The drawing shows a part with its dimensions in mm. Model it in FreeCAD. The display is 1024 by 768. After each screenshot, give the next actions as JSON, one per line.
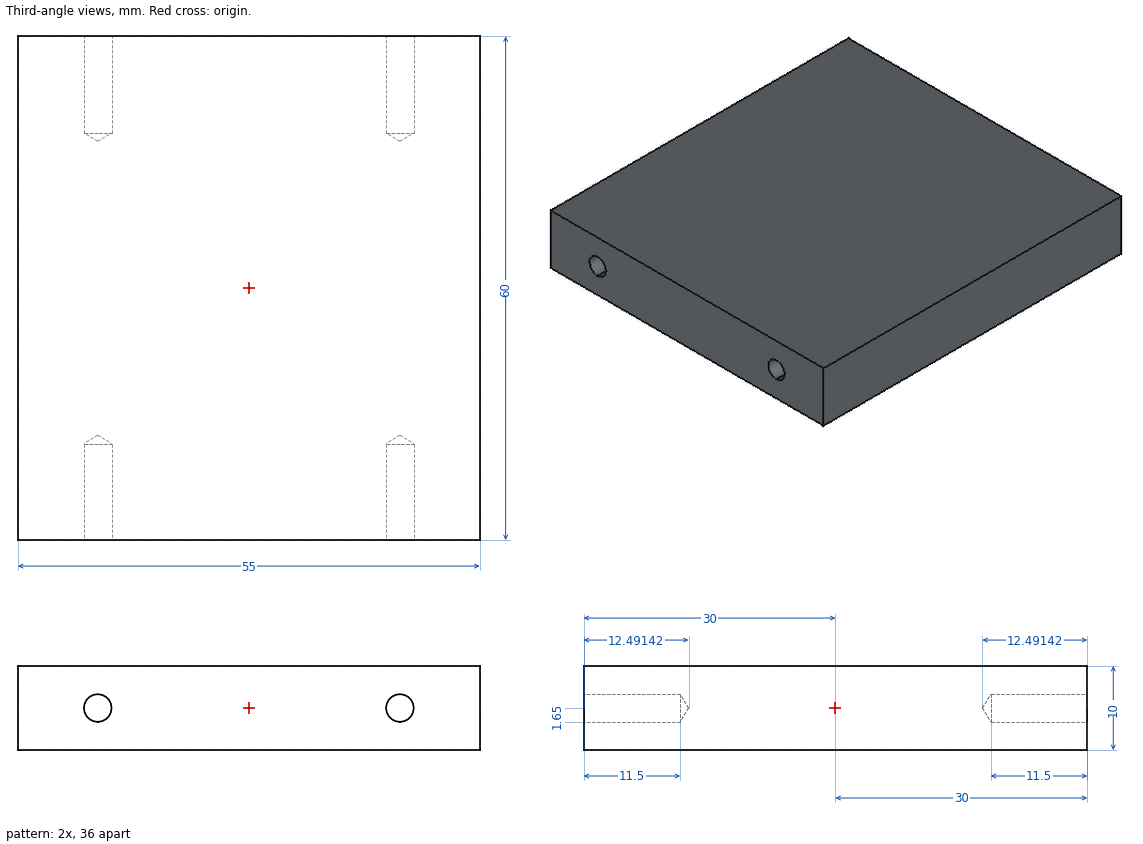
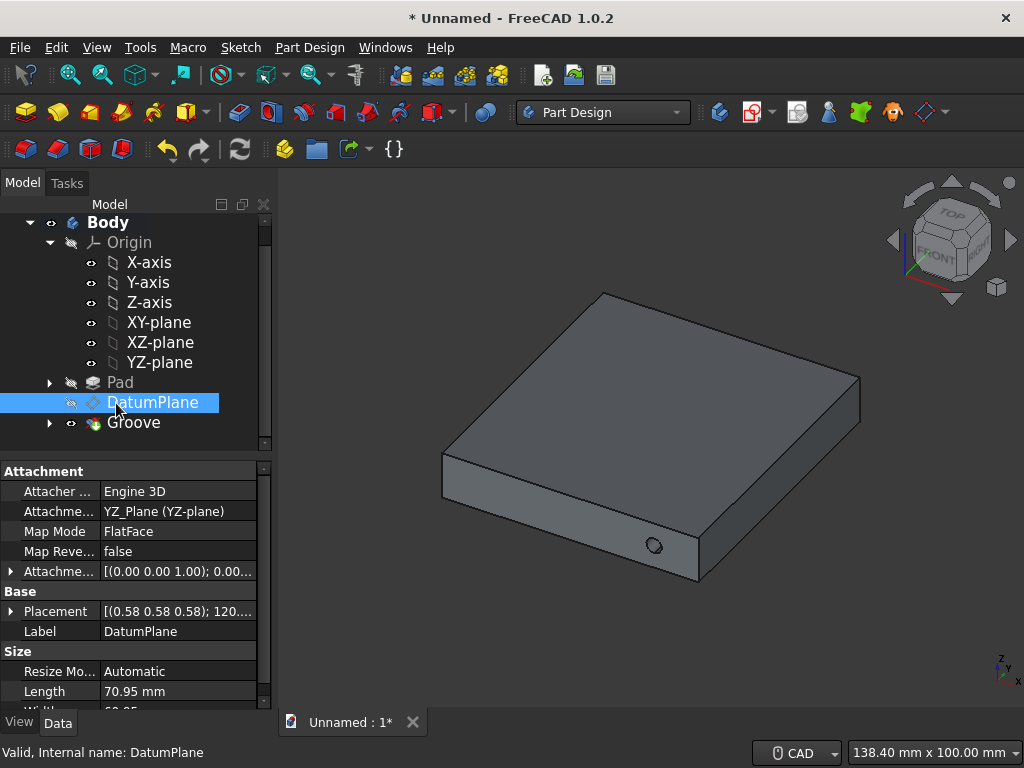
{"action": "left_click", "coordinate": [116, 423]}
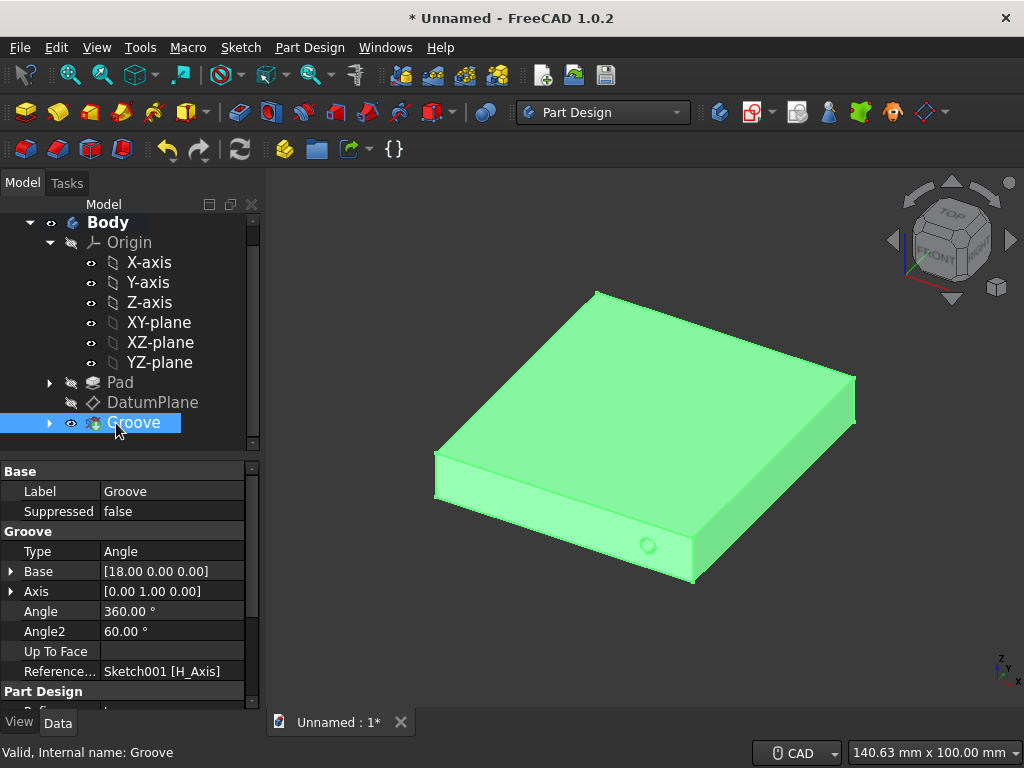
{"action": "left_click", "coordinate": [434, 76]}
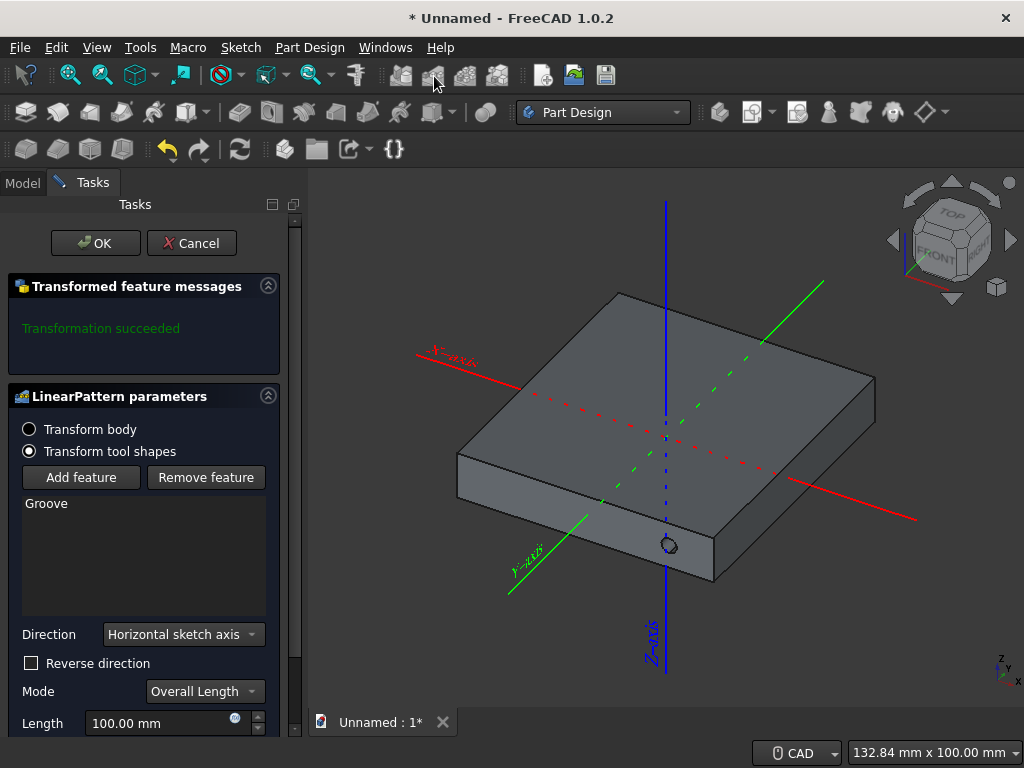
{"action": "left_click", "coordinate": [184, 634]}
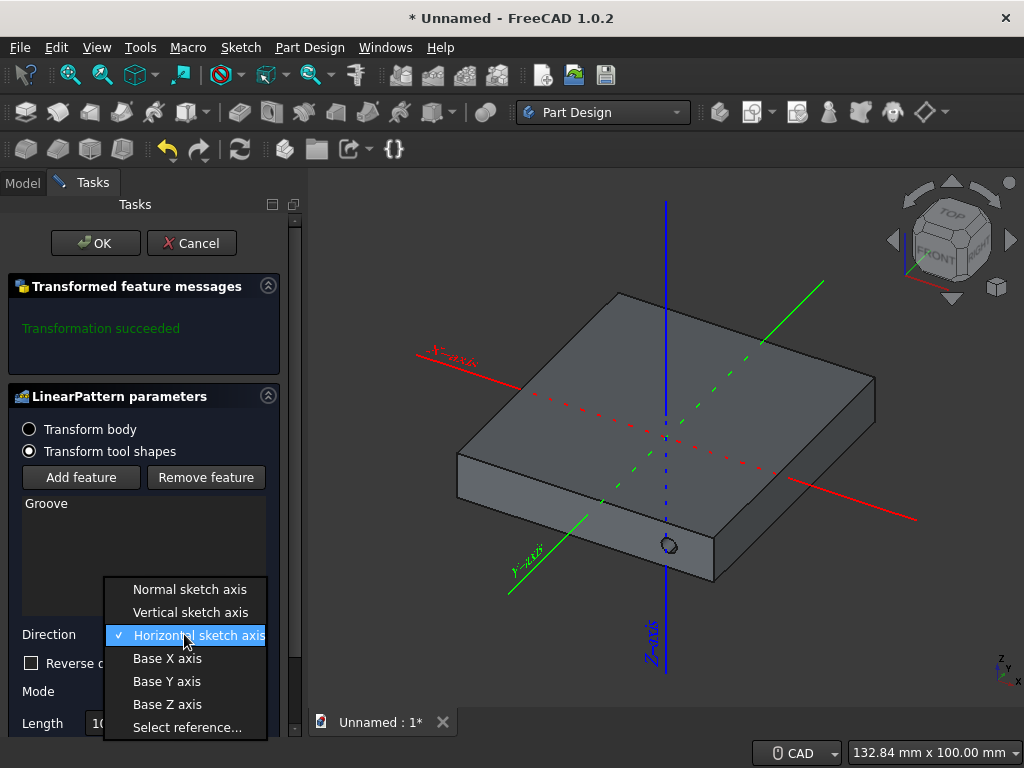
{"action": "left_click", "coordinate": [184, 658]}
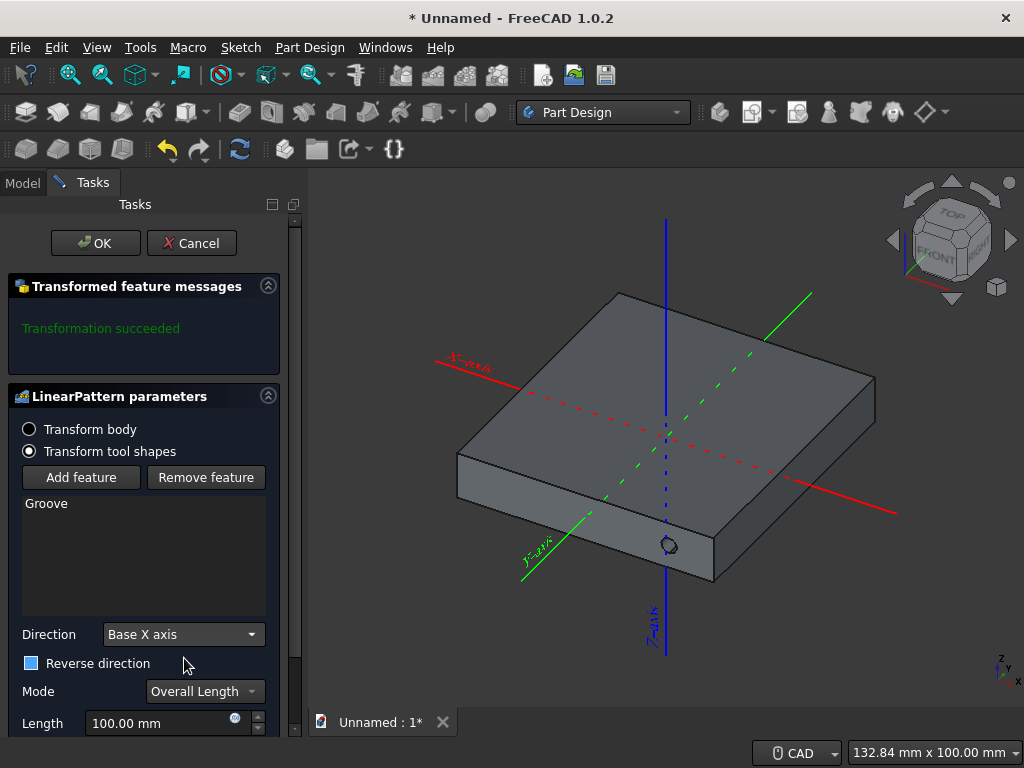
{"action": "left_click", "coordinate": [206, 692]}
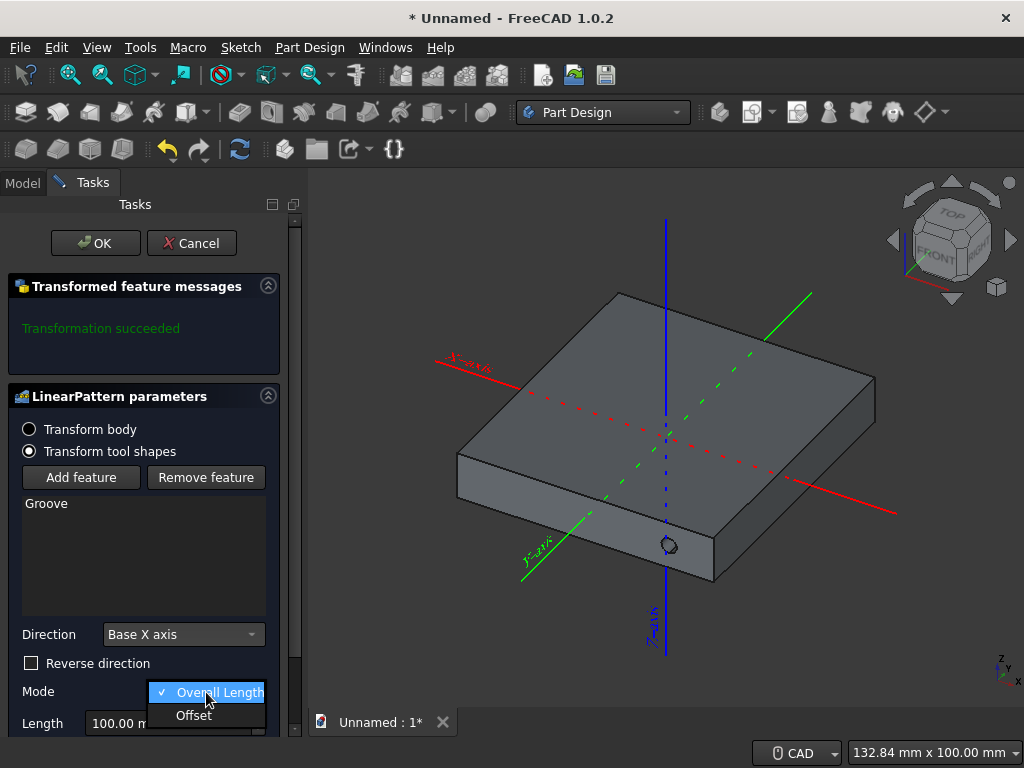
{"action": "left_click", "coordinate": [206, 716]}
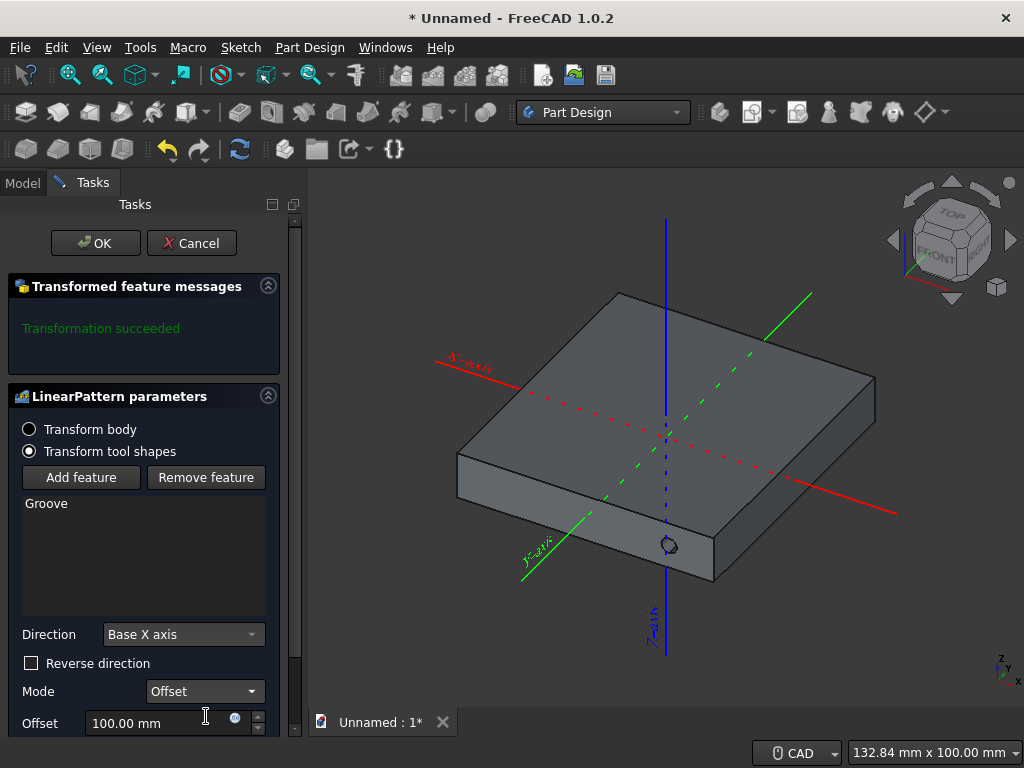
{"action": "triple_click", "coordinate": [168, 723]}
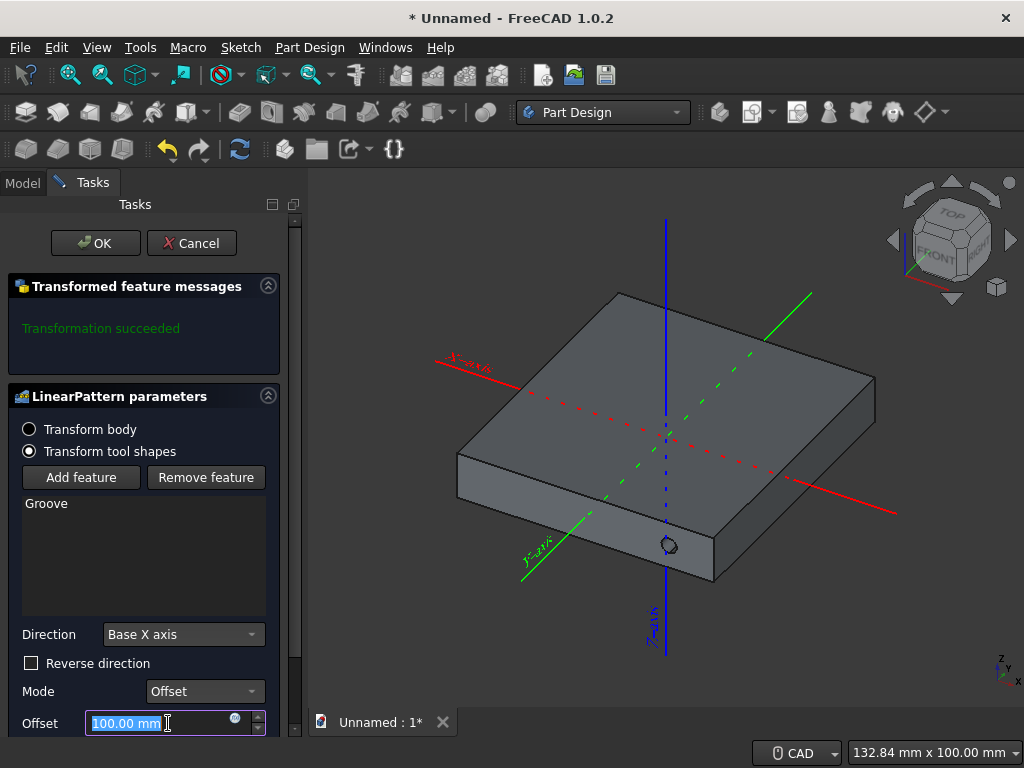
{"action": "type", "text": "36"}
{"action": "key", "text": "Tab"}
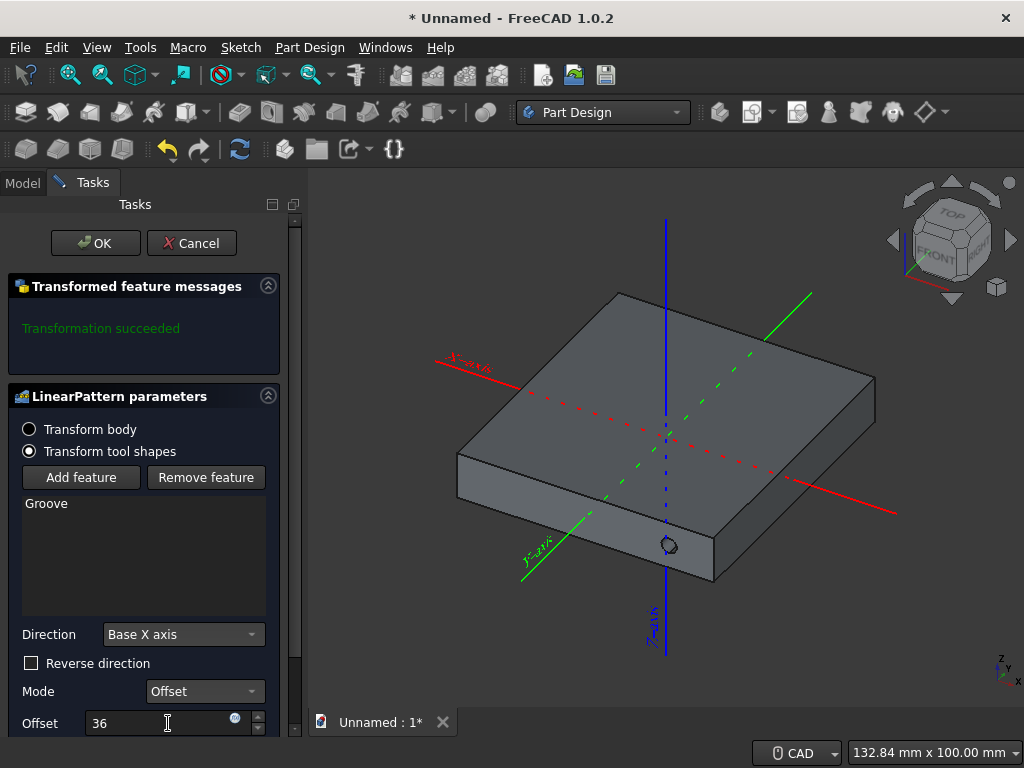
{"action": "scroll", "coordinate": [295, 475], "scroll_direction": "down", "scroll_amount": 2}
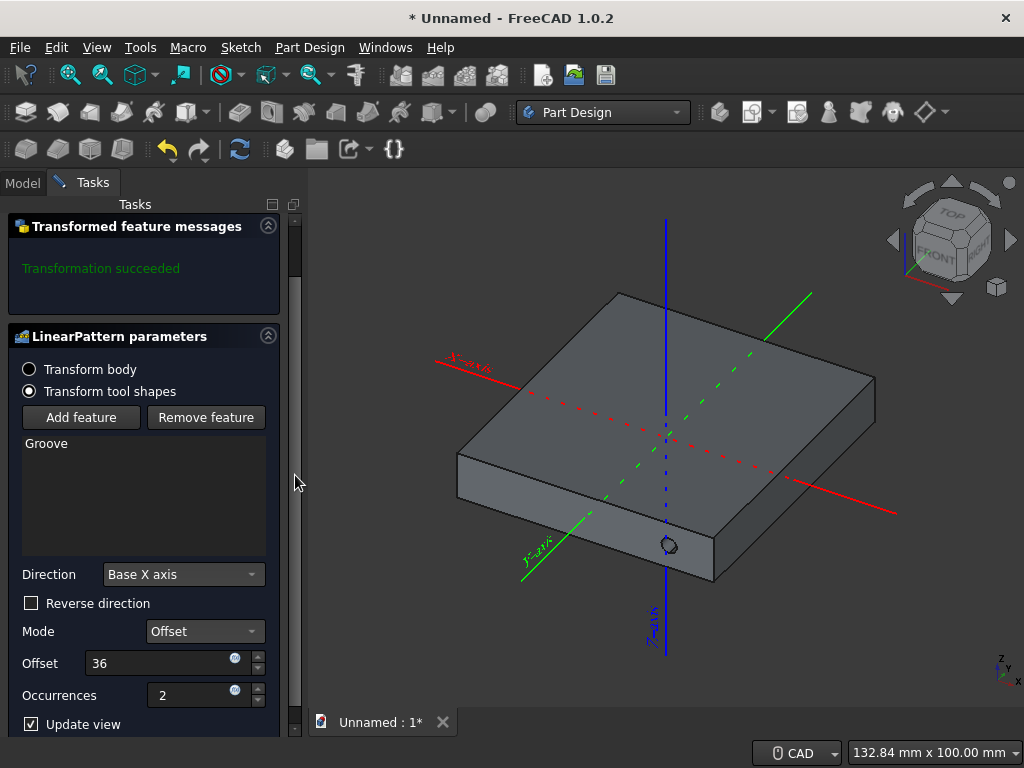
{"action": "triple_click", "coordinate": [198, 676]}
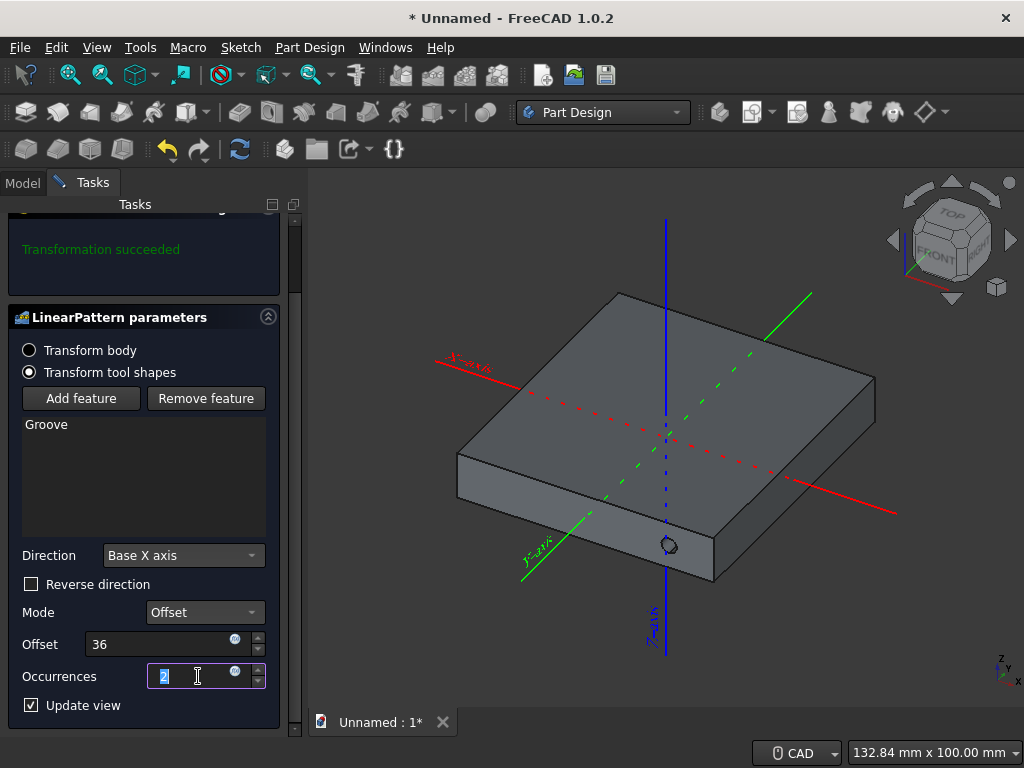
{"action": "type", "text": "2"}
{"action": "key", "text": "Tab"}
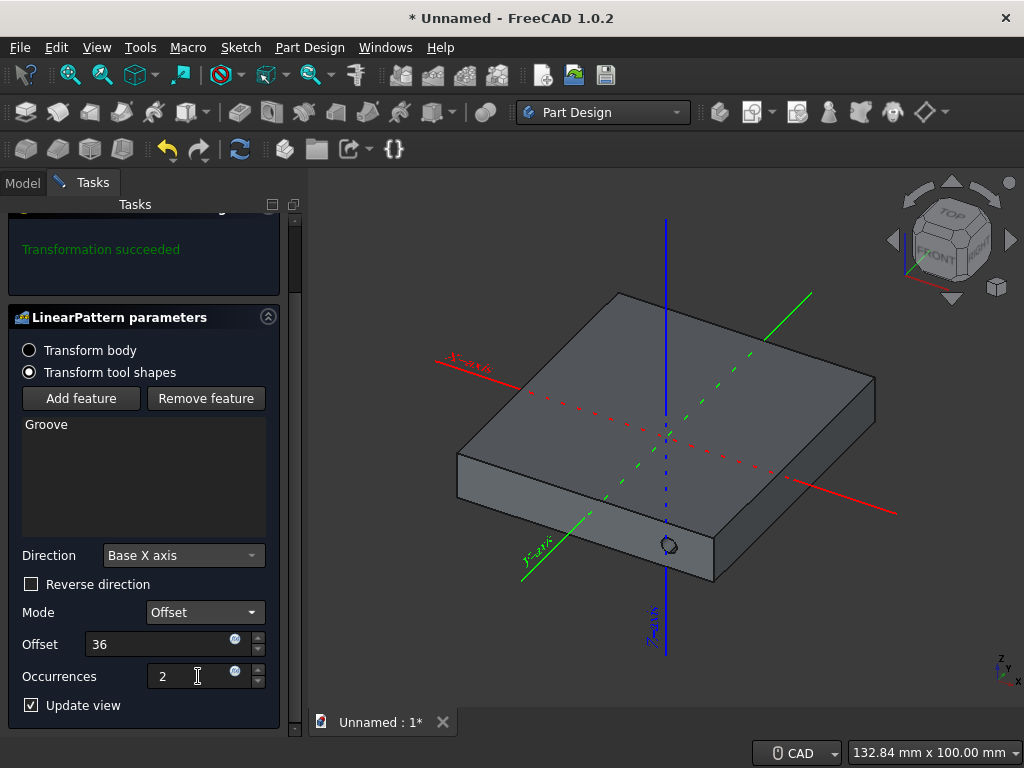
{"action": "left_click", "coordinate": [30, 584]}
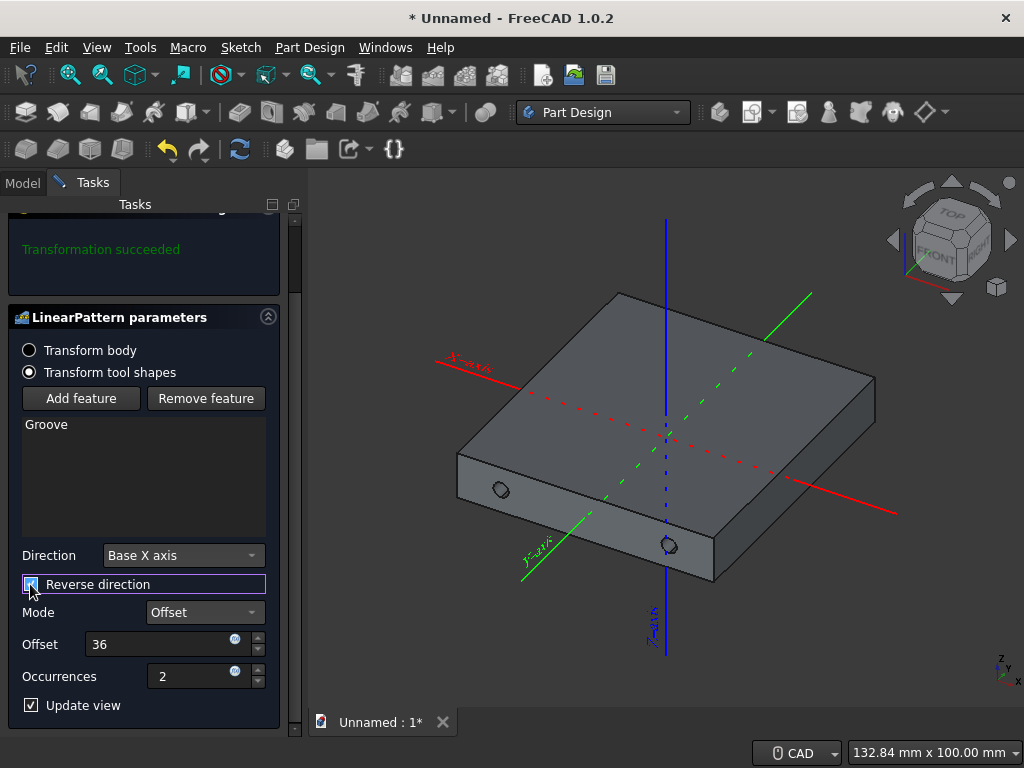
{"action": "scroll", "coordinate": [295, 475], "scroll_direction": "up", "scroll_amount": 3}